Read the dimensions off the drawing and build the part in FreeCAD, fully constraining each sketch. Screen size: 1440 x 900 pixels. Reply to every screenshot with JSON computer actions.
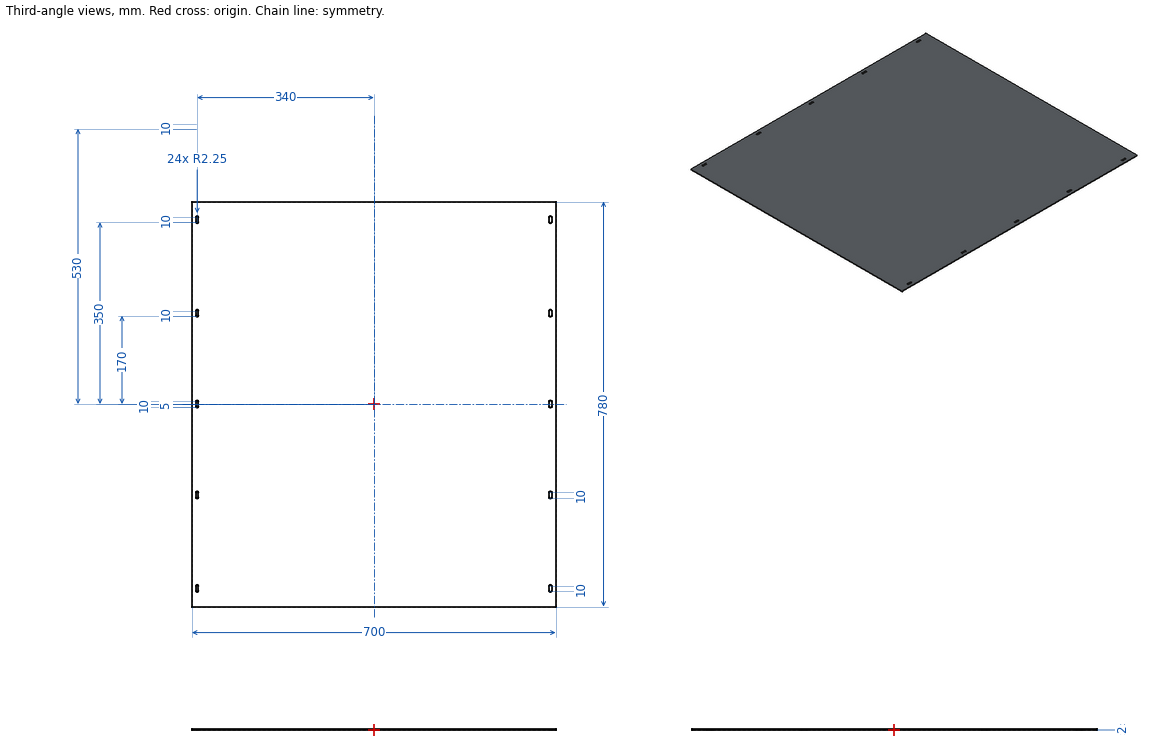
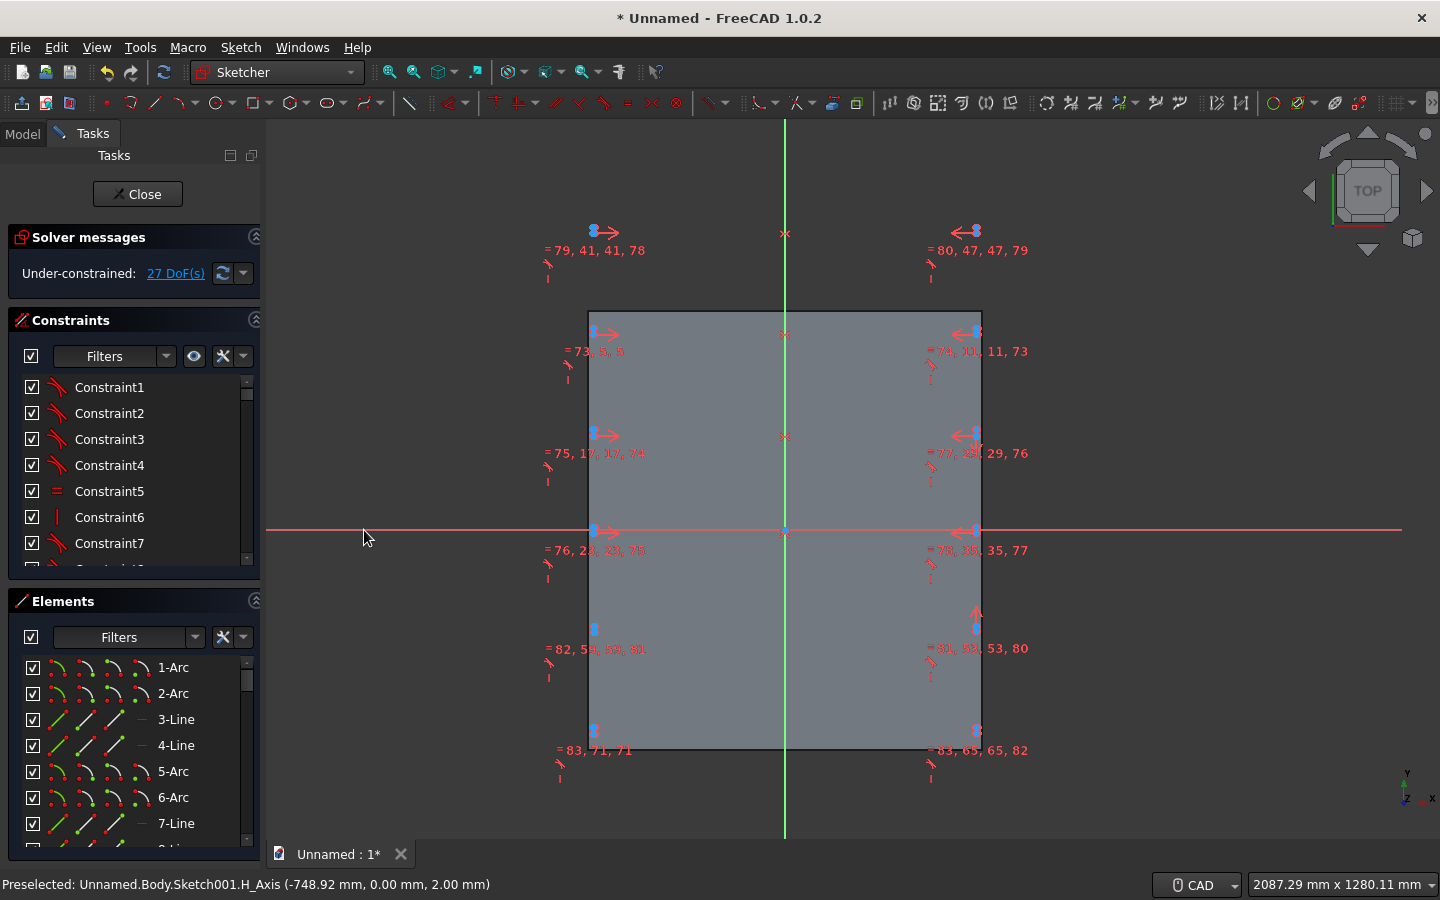
{"action": "scroll", "coordinate": [594, 430], "scroll_direction": "up", "scroll_amount": 12}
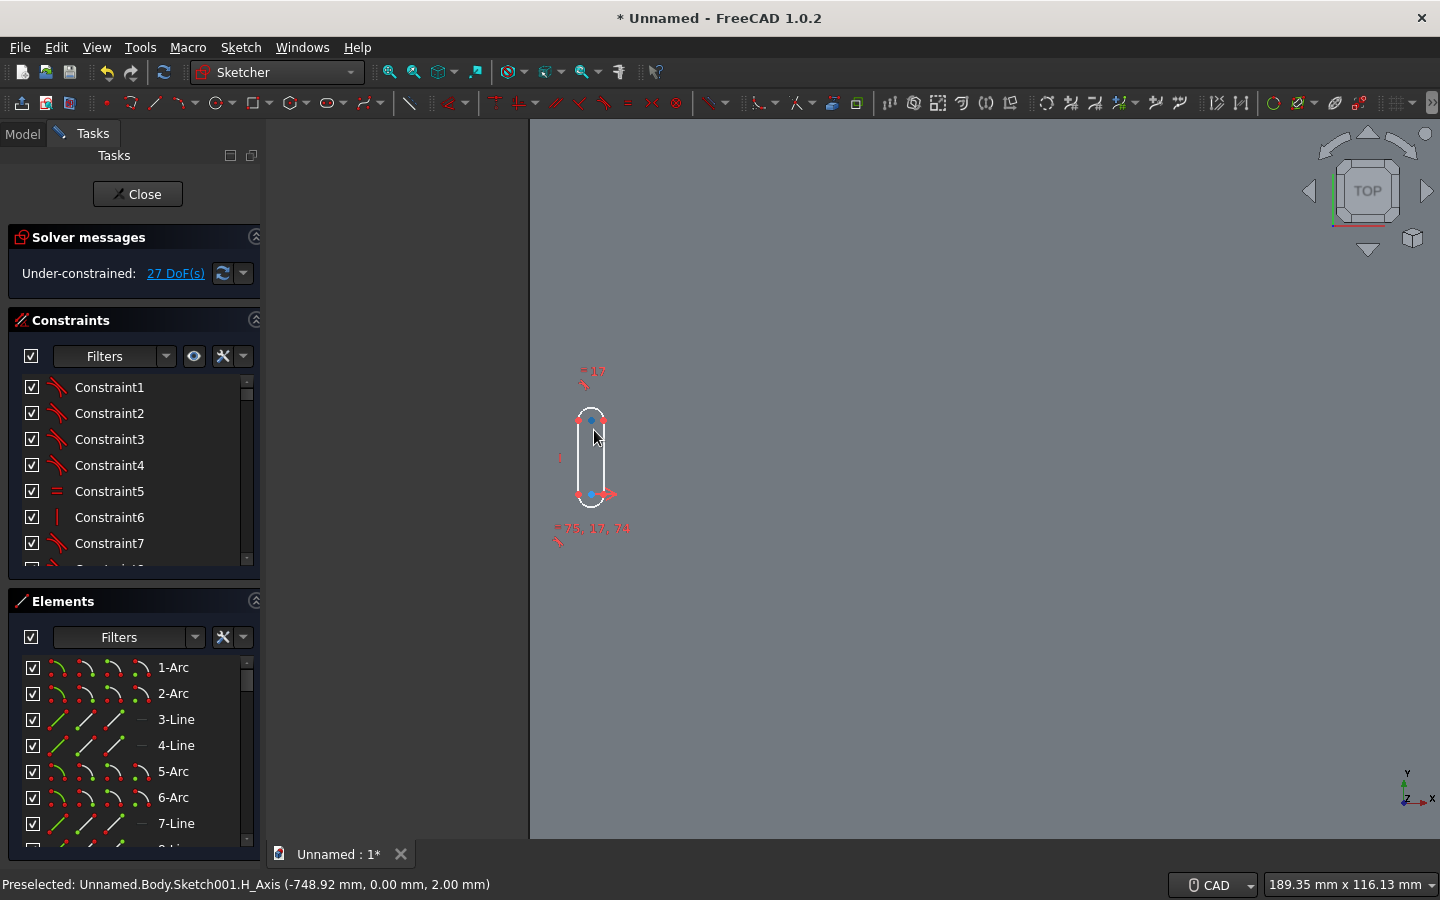
{"action": "left_click", "coordinate": [591, 421]}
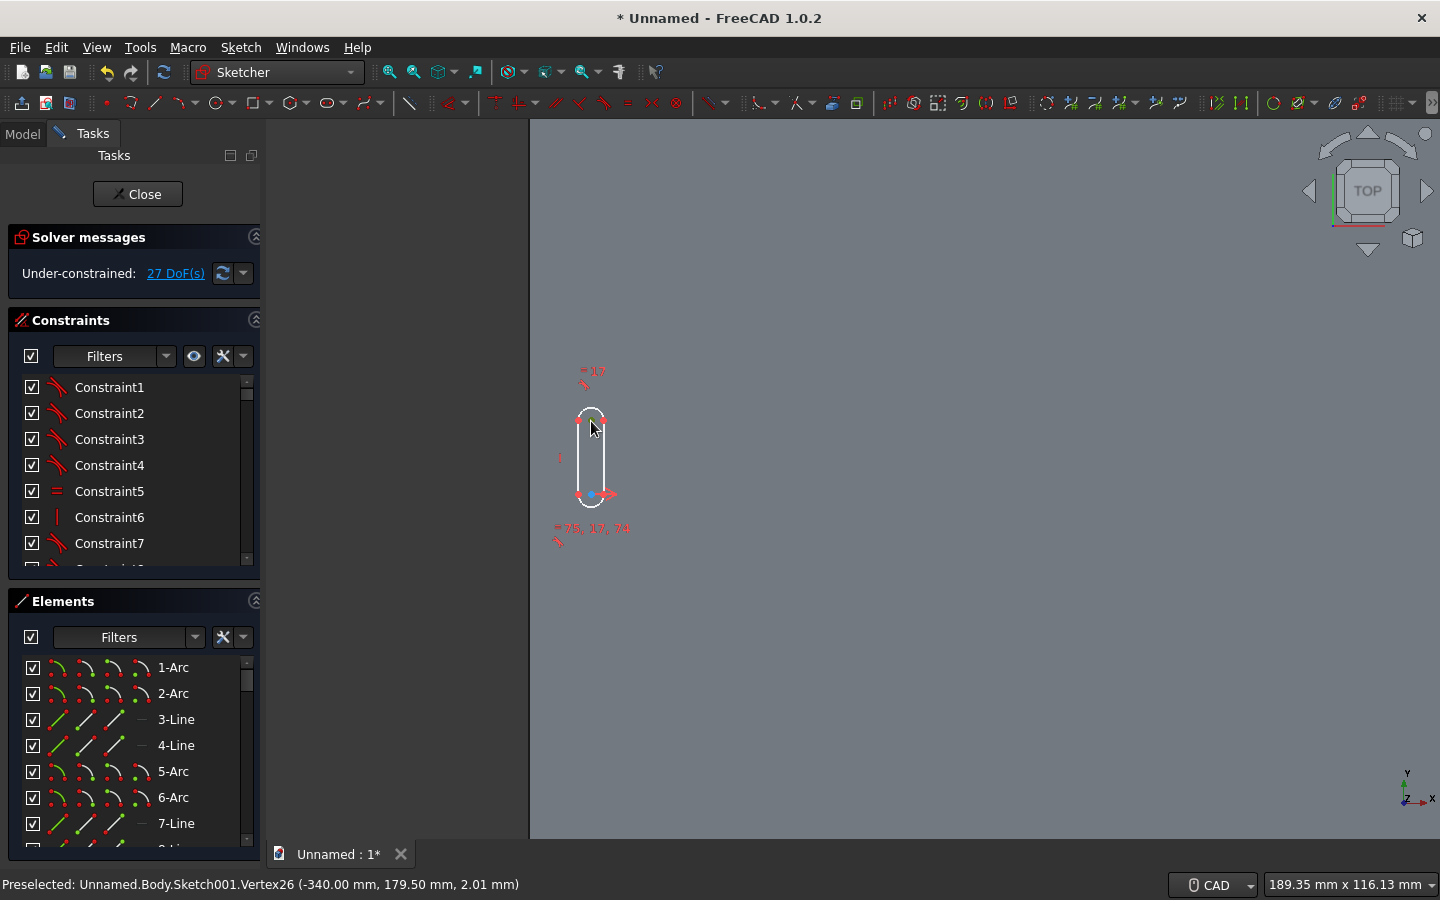
{"action": "scroll", "coordinate": [593, 429], "scroll_direction": "down", "scroll_amount": 12}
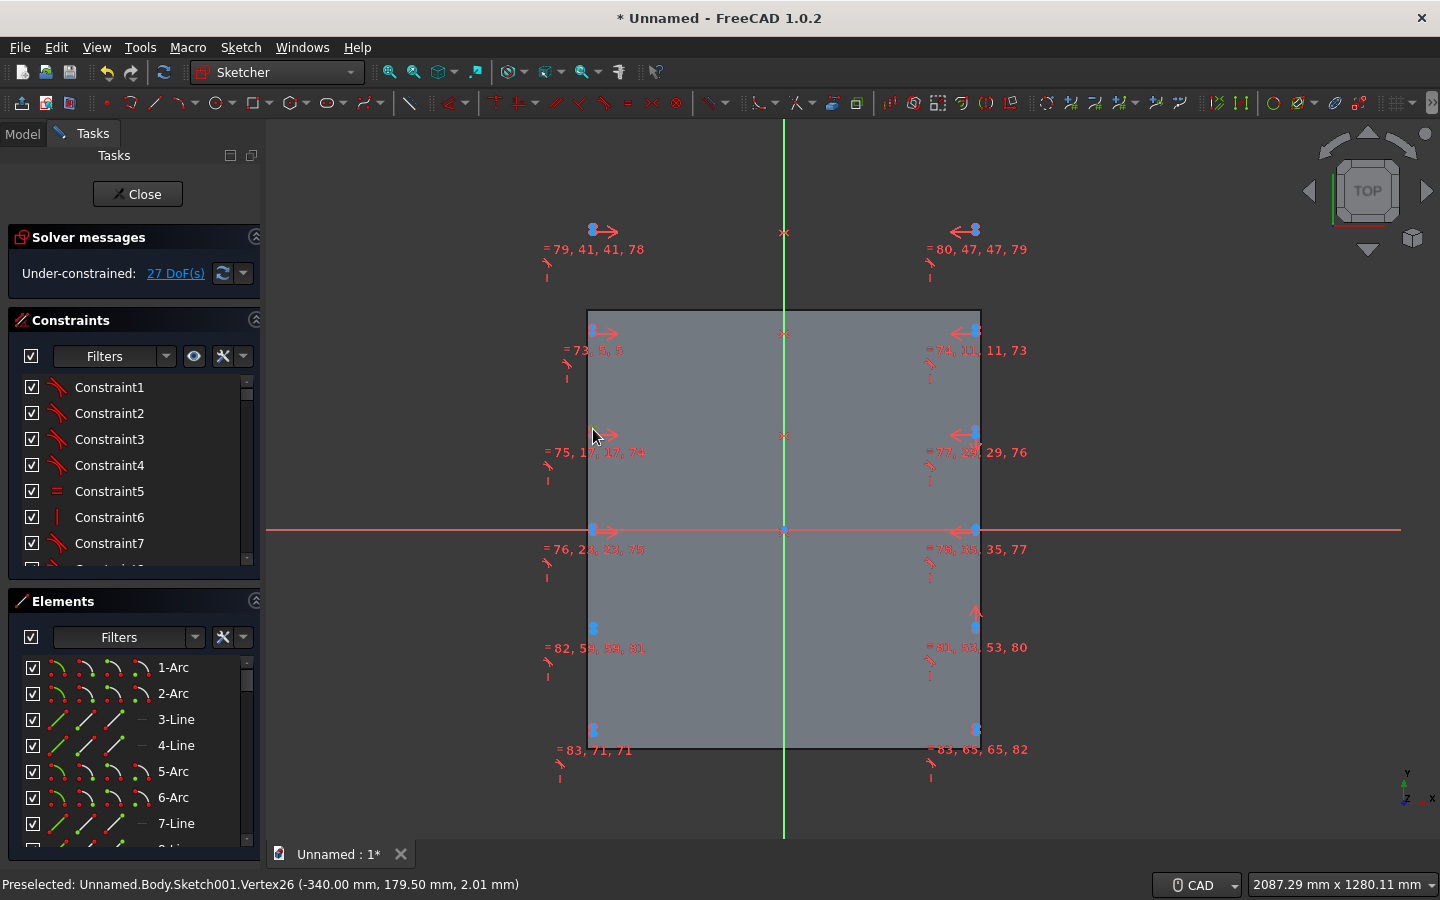
{"action": "scroll", "coordinate": [593, 632], "scroll_direction": "up", "scroll_amount": 12}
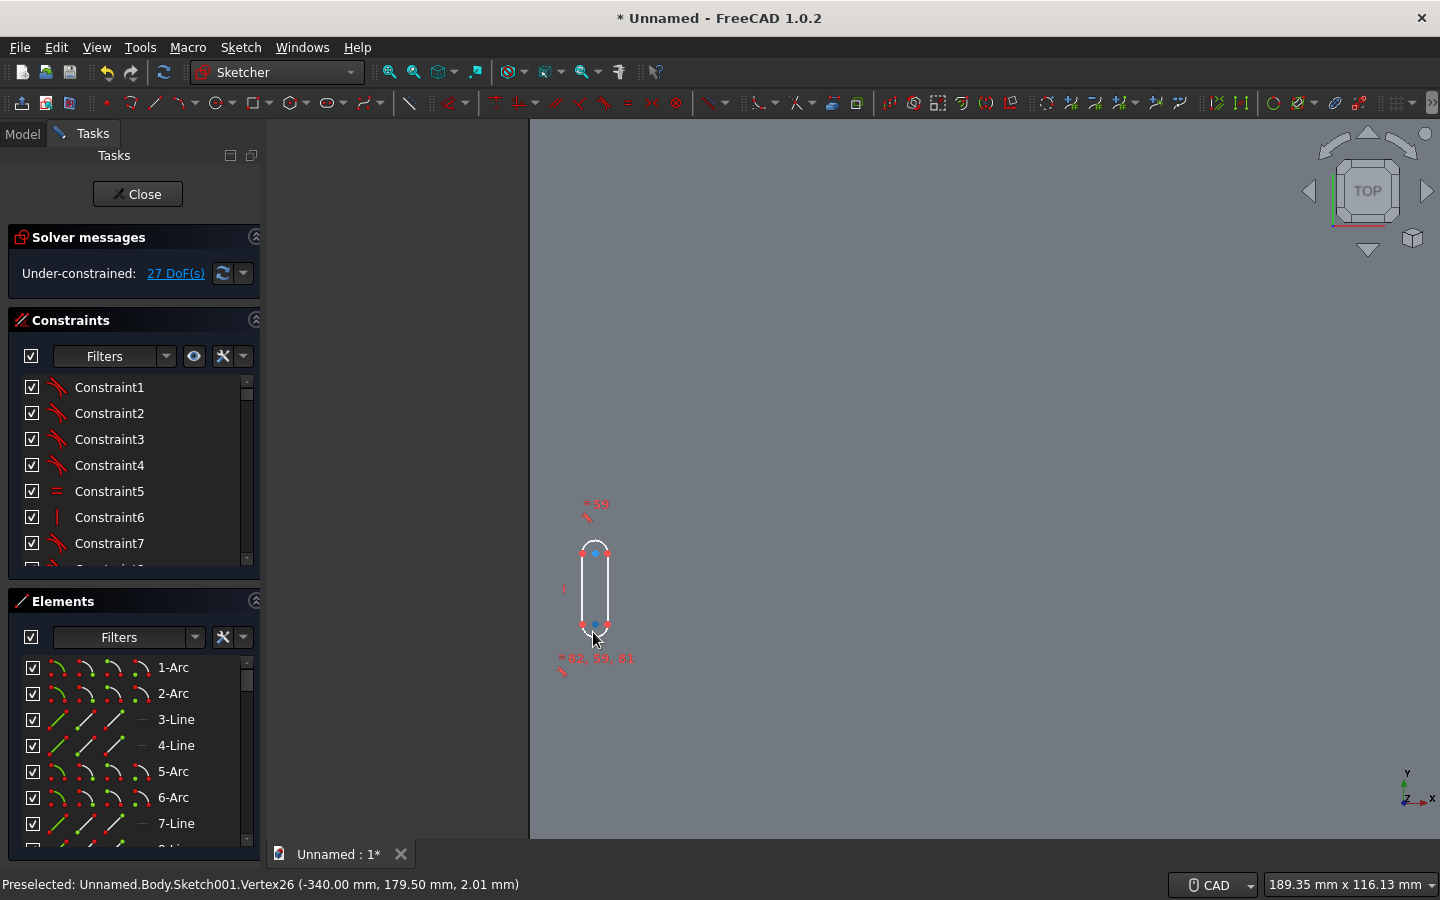
{"action": "left_click", "coordinate": [595, 624]}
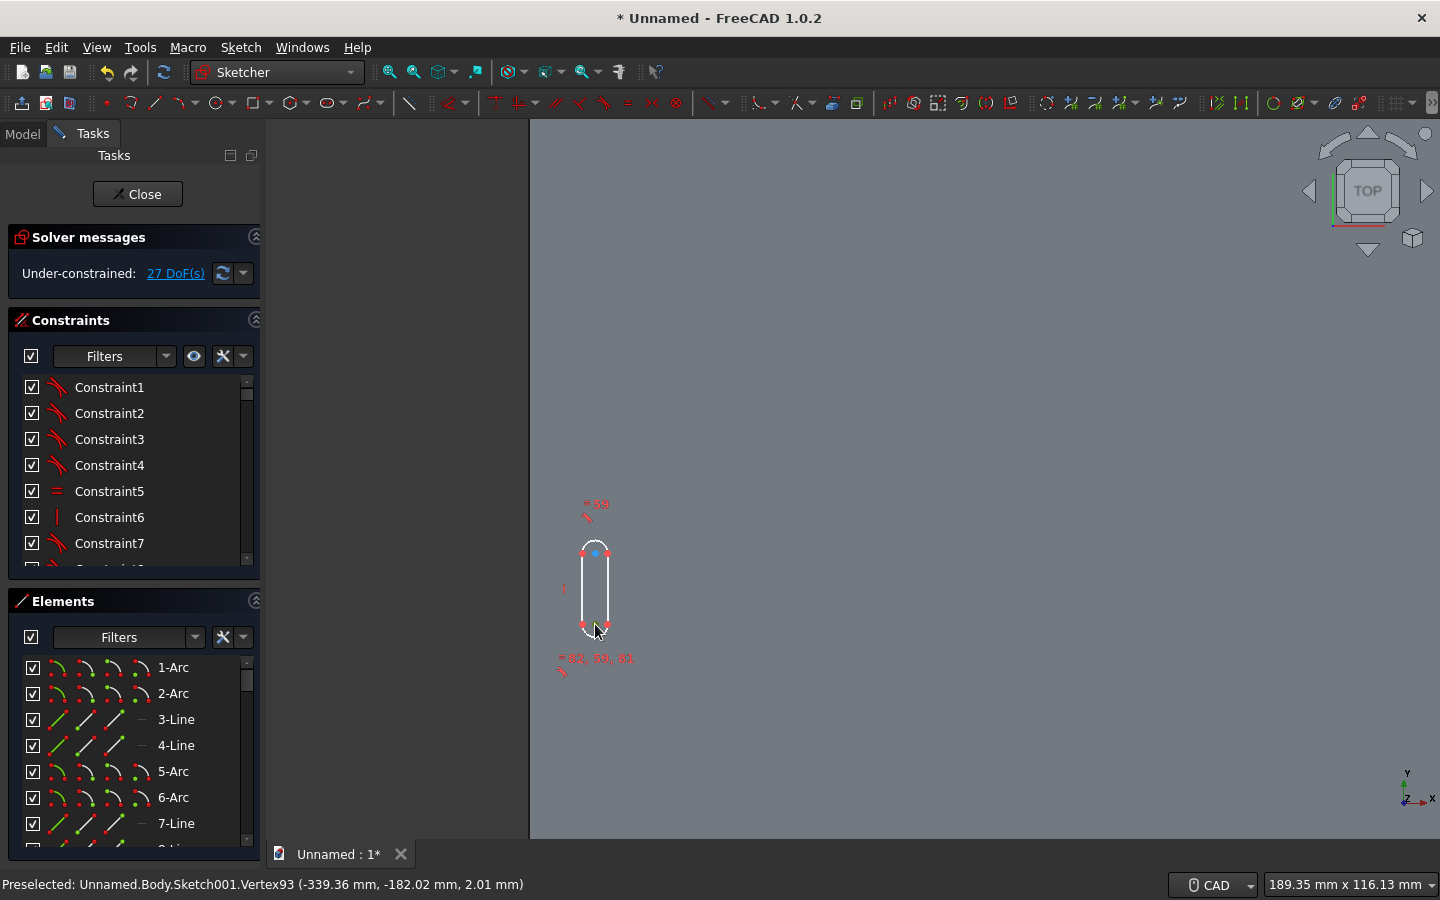
{"action": "scroll", "coordinate": [593, 633], "scroll_direction": "down", "scroll_amount": 12}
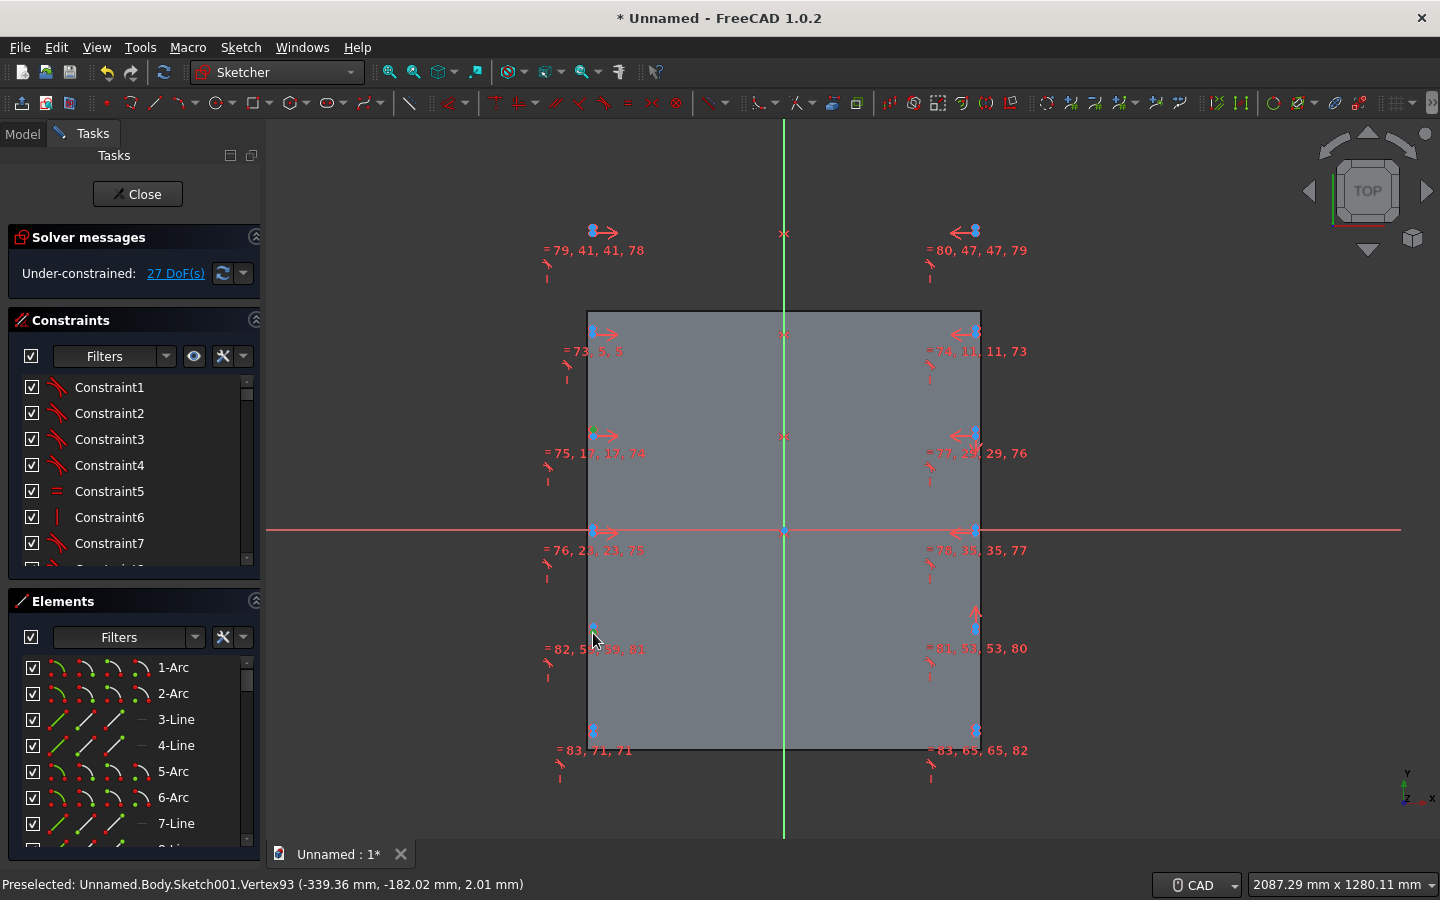
{"action": "left_click", "coordinate": [364, 530]}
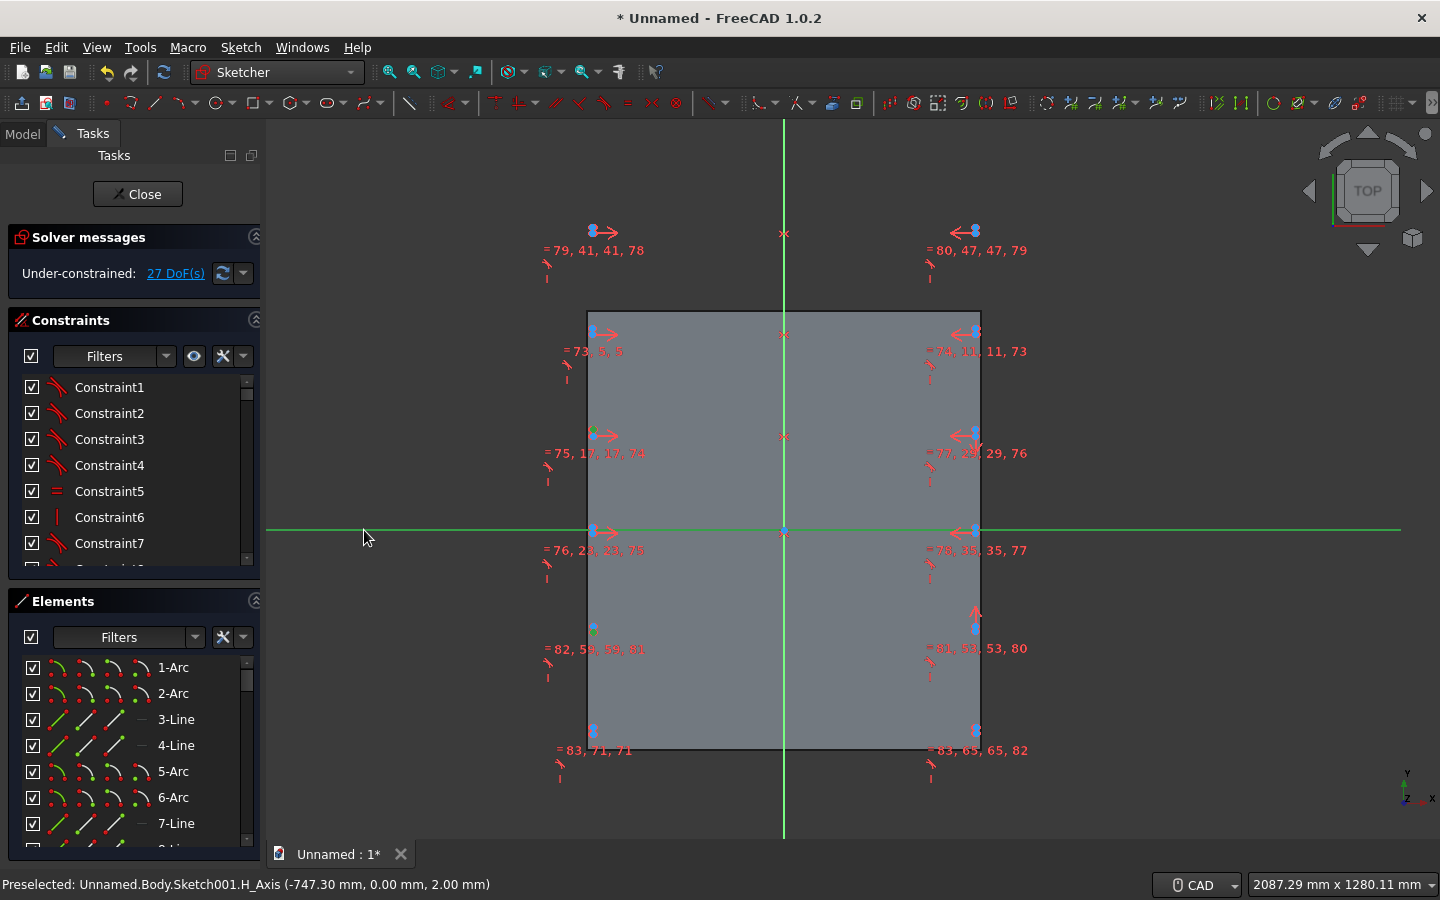
{"action": "key", "text": "s"}